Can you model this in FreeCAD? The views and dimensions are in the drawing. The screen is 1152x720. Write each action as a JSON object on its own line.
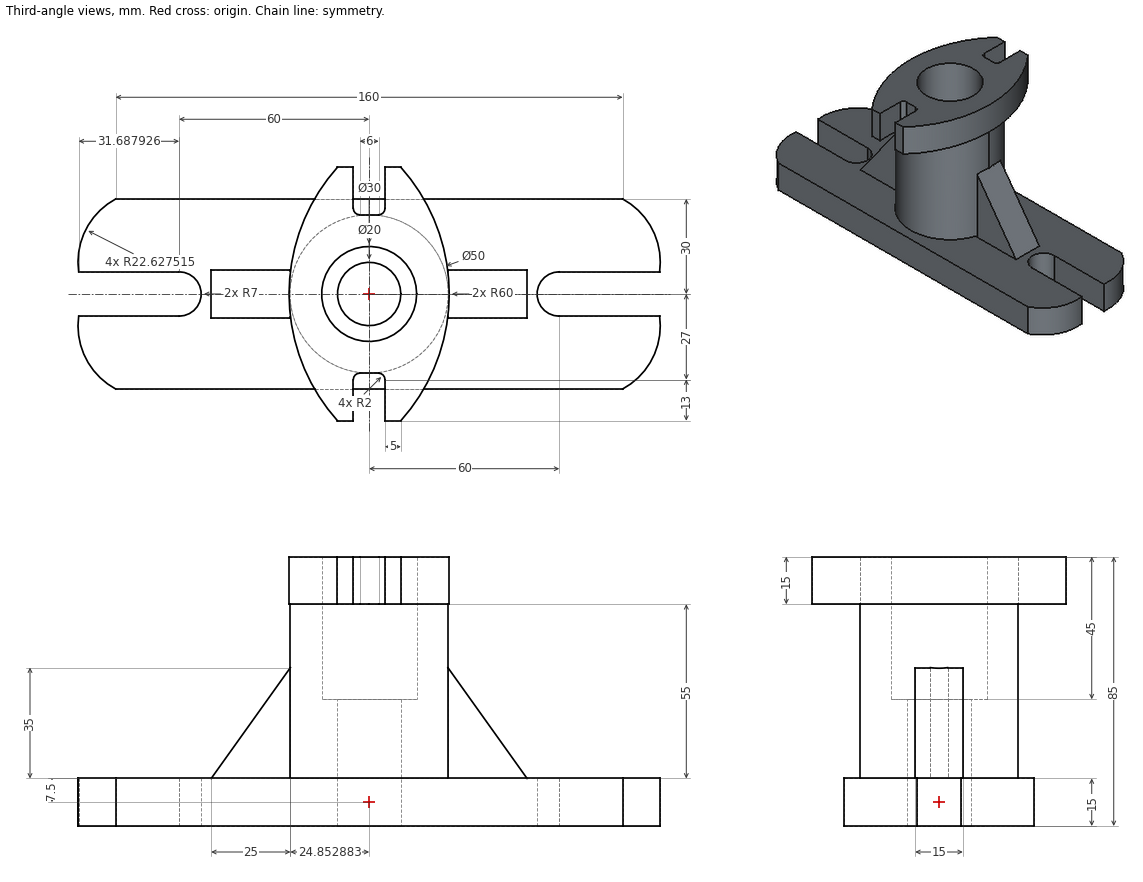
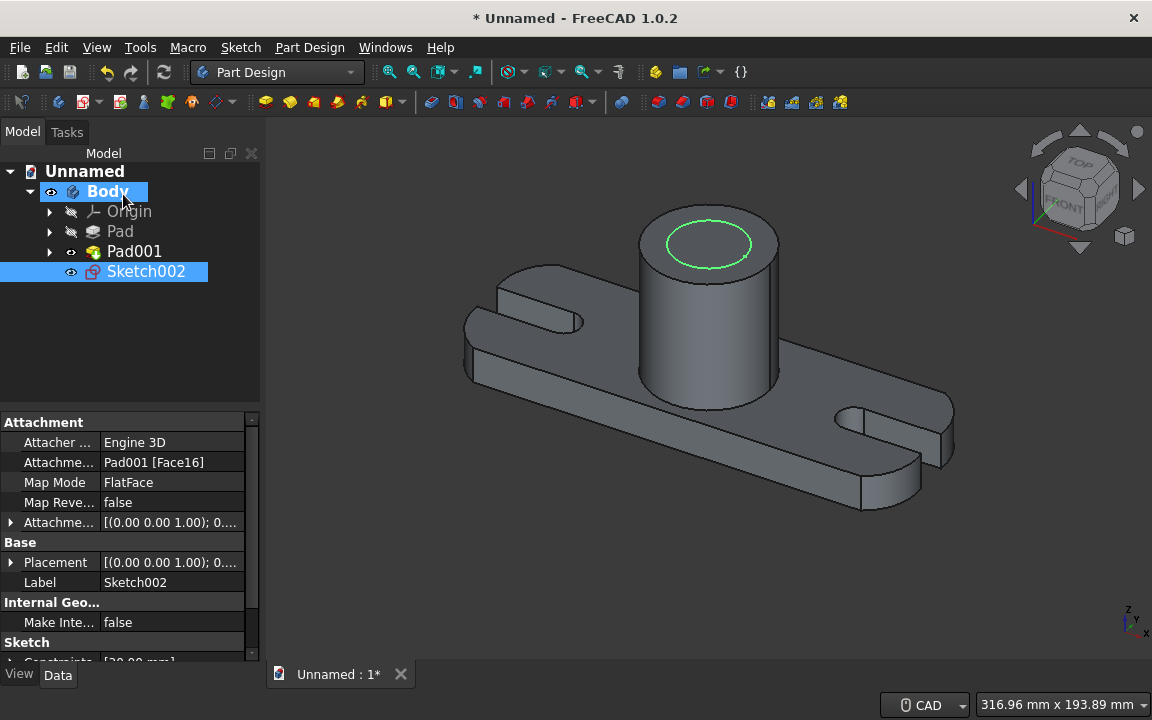
{"action": "left_click", "coordinate": [432, 102]}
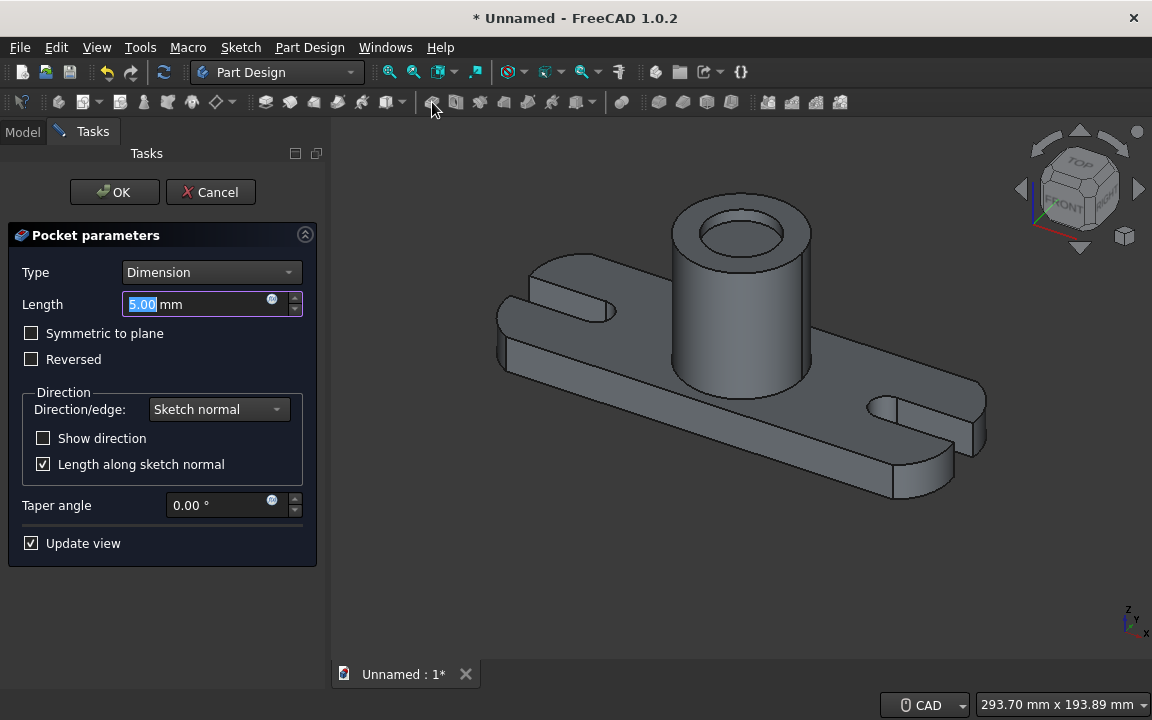
{"action": "left_click", "coordinate": [212, 272]}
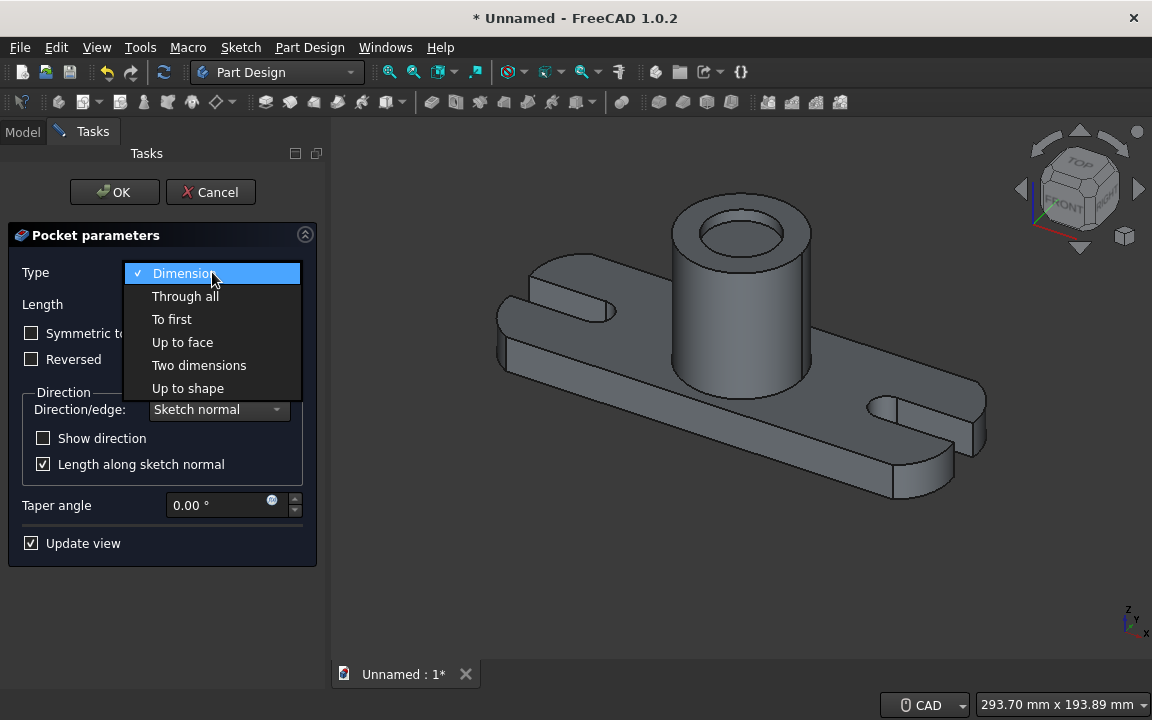
{"action": "left_click", "coordinate": [212, 296]}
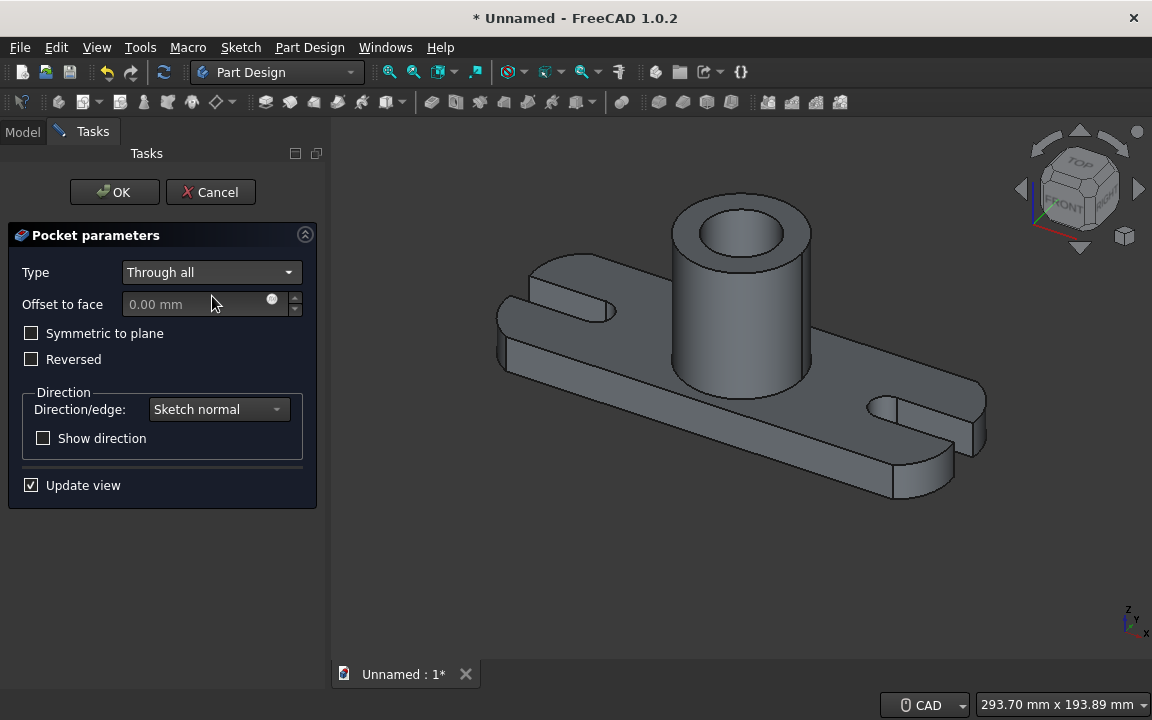
{"action": "left_click", "coordinate": [115, 192]}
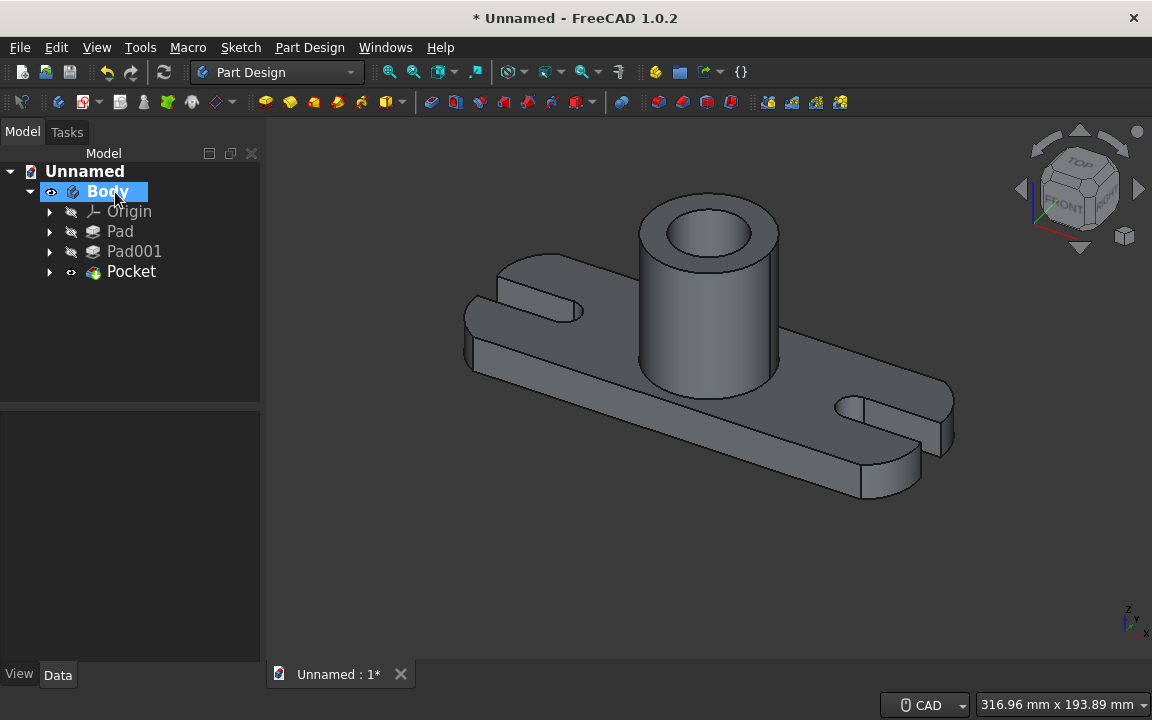
{"action": "left_click", "coordinate": [50, 212]}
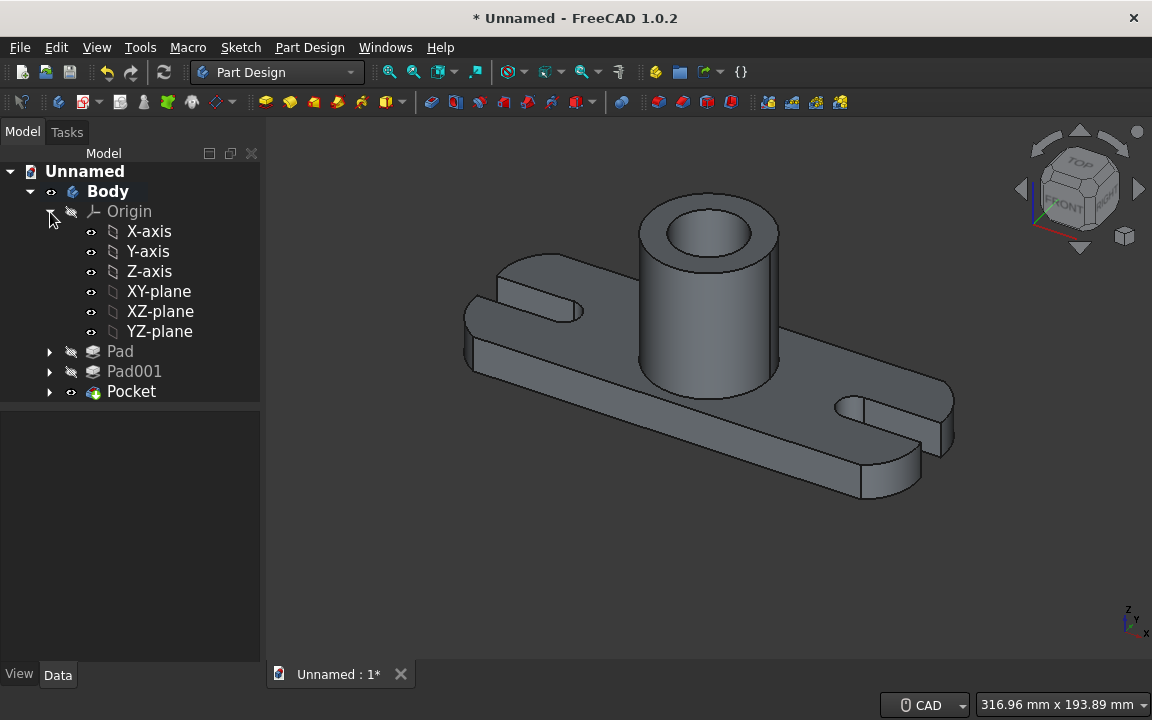
{"action": "left_click", "coordinate": [136, 292]}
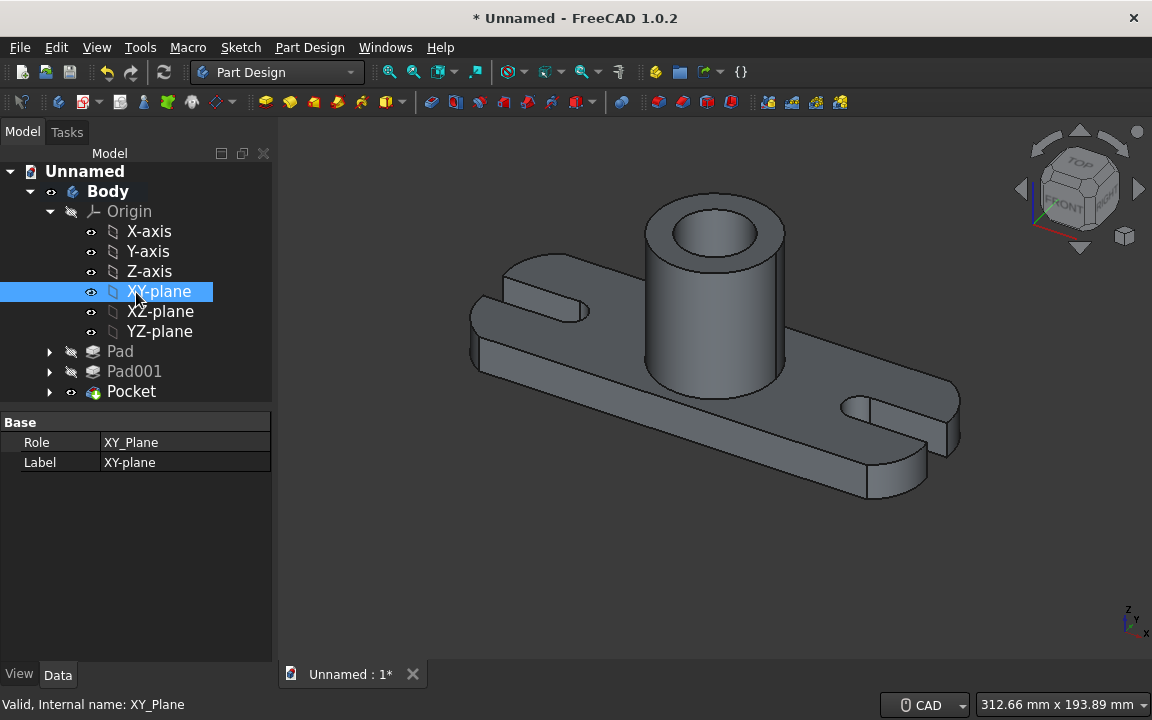
{"action": "left_click", "coordinate": [216, 102]}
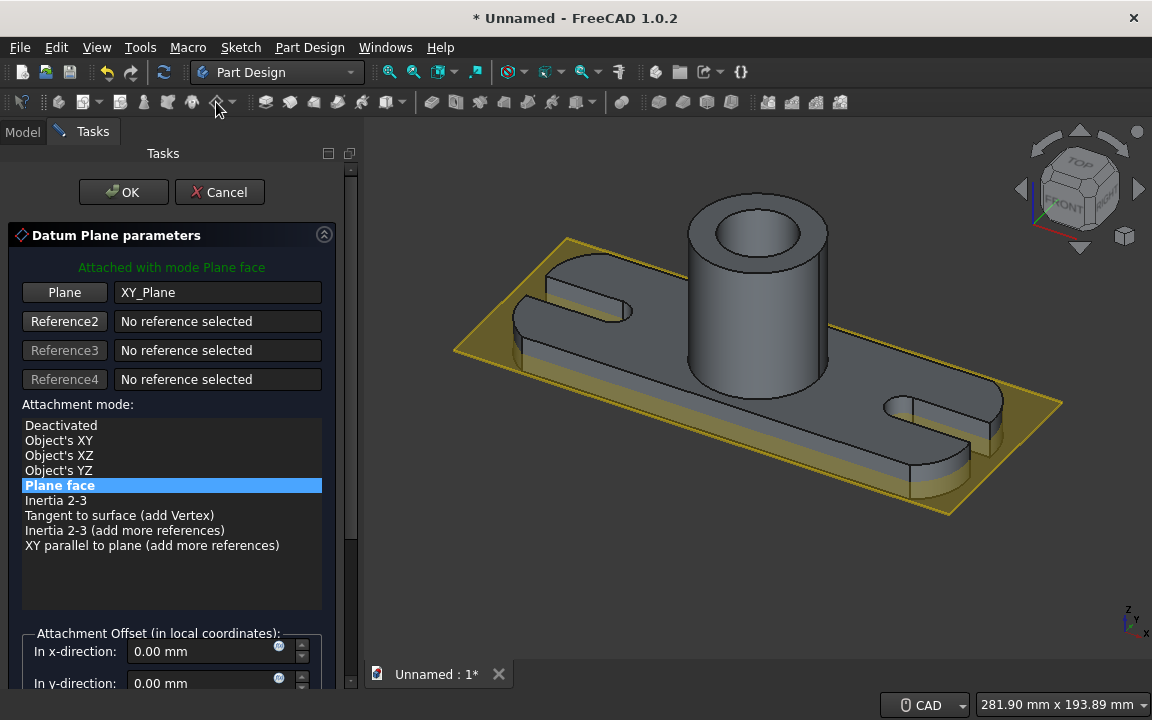
{"action": "scroll", "coordinate": [351, 426], "scroll_direction": "down", "scroll_amount": 2}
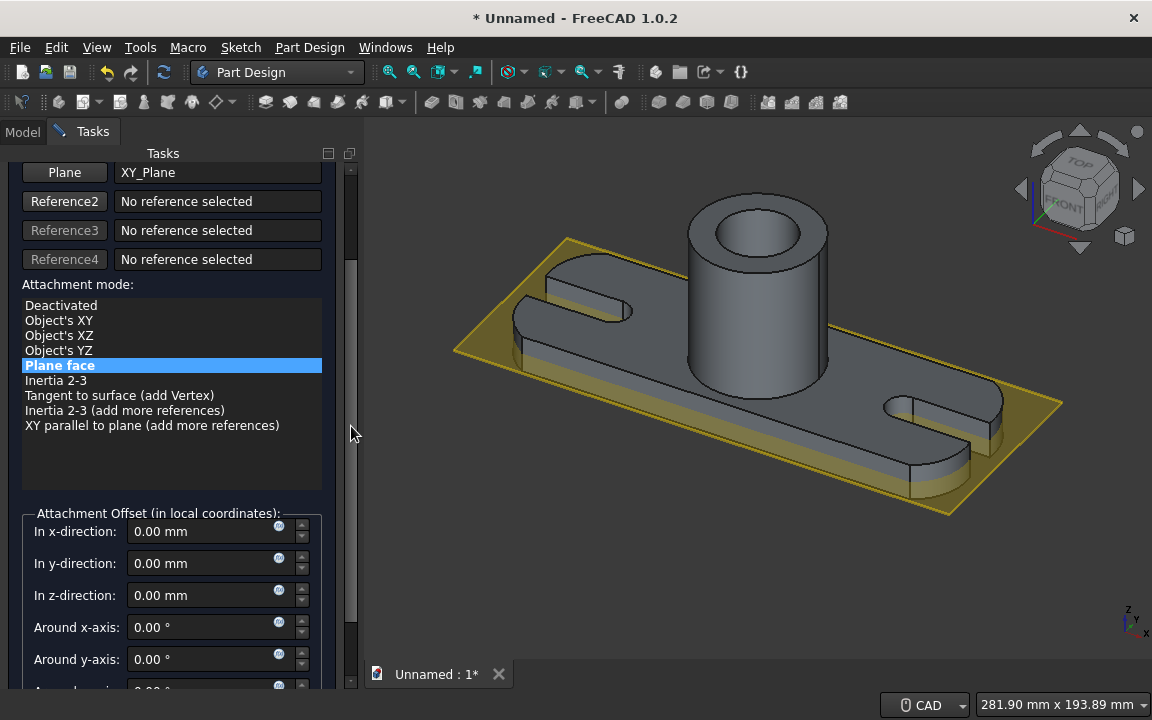
{"action": "triple_click", "coordinate": [210, 595]}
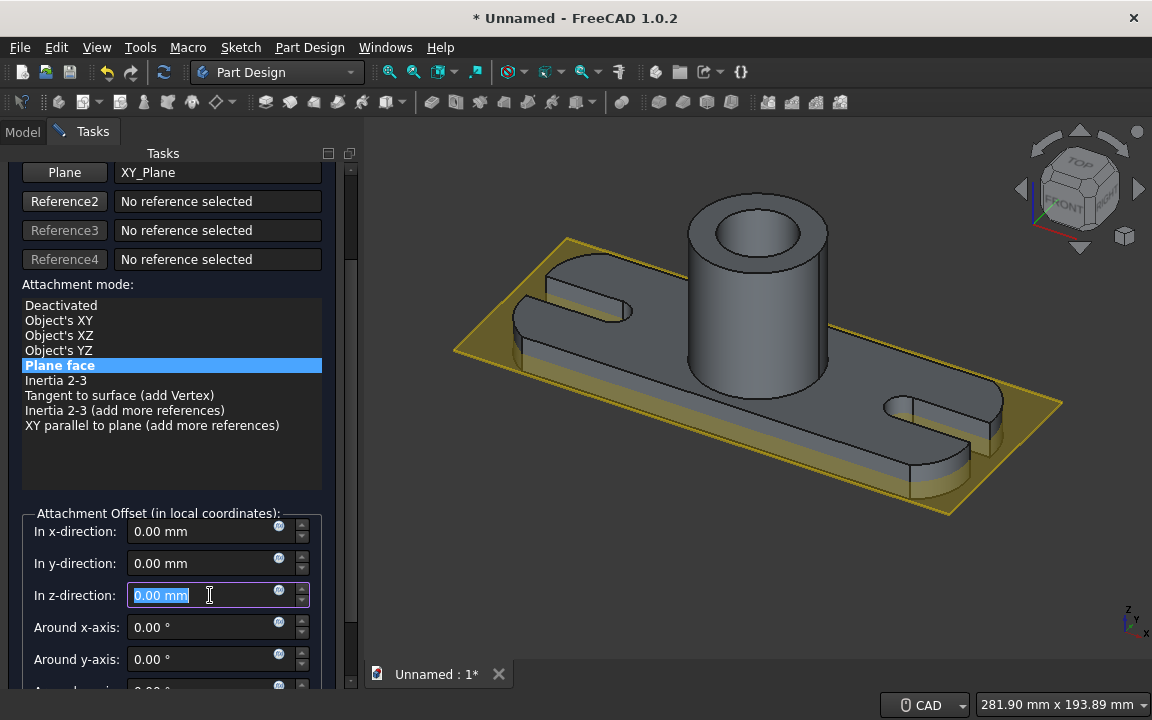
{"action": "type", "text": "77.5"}
{"action": "key", "text": "Tab"}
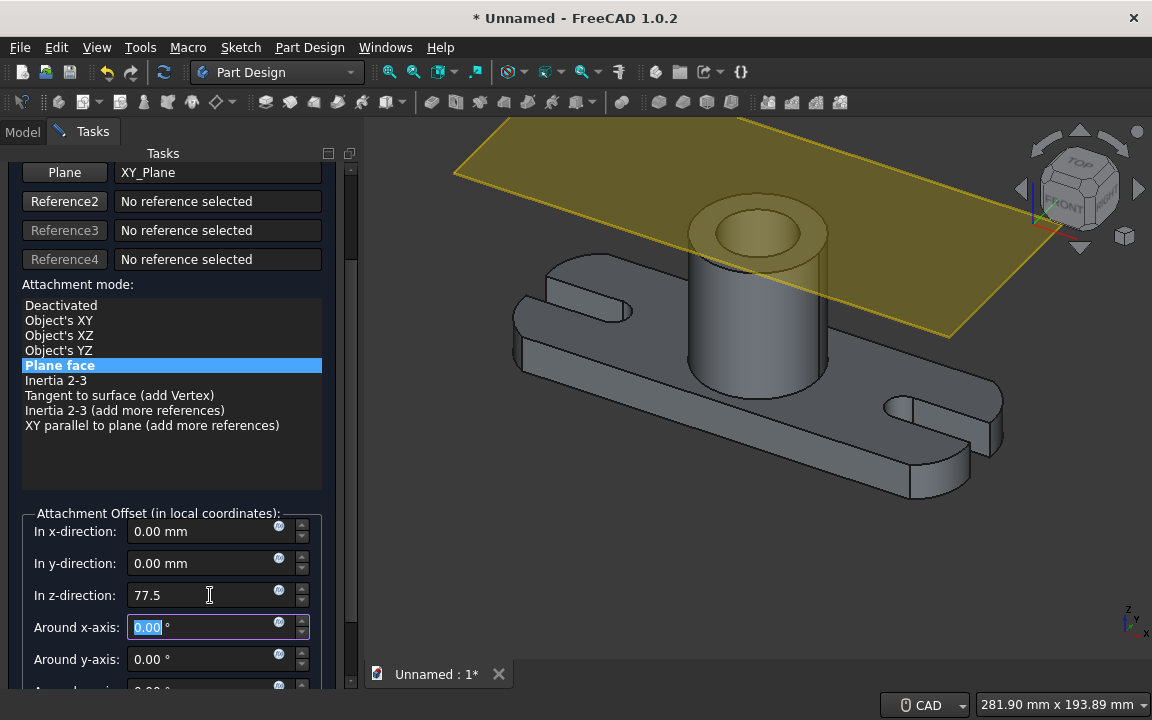
{"action": "scroll", "coordinate": [351, 426], "scroll_direction": "up", "scroll_amount": 3}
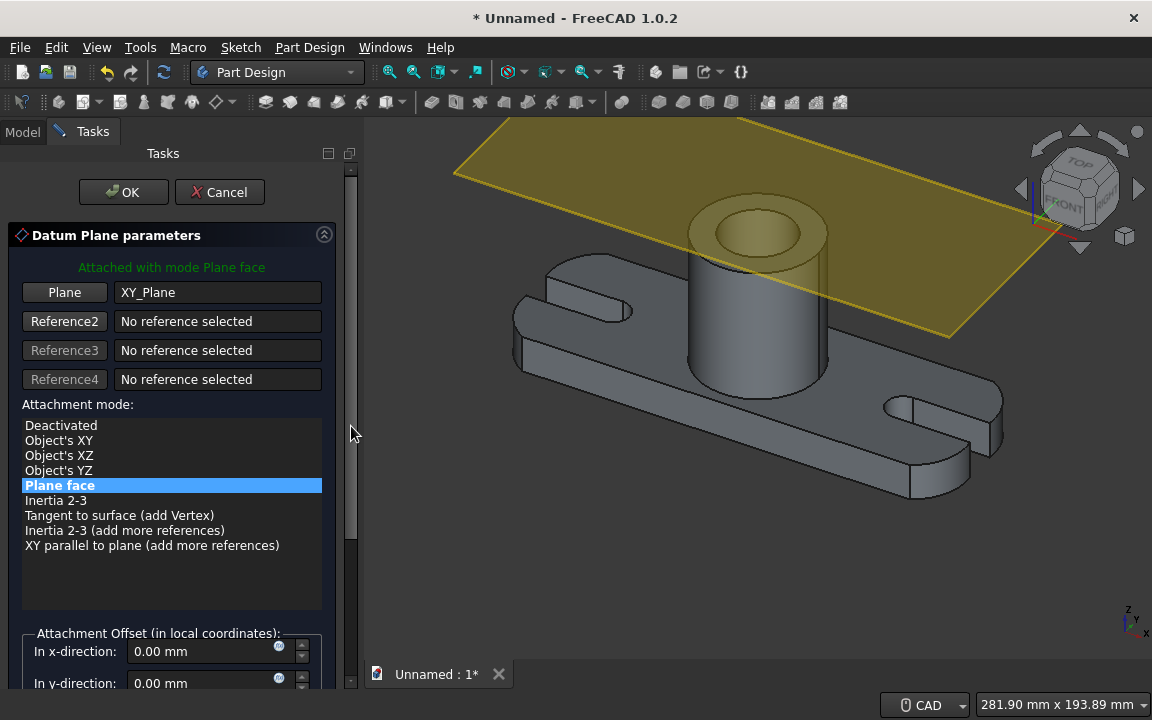
{"action": "left_click", "coordinate": [124, 192]}